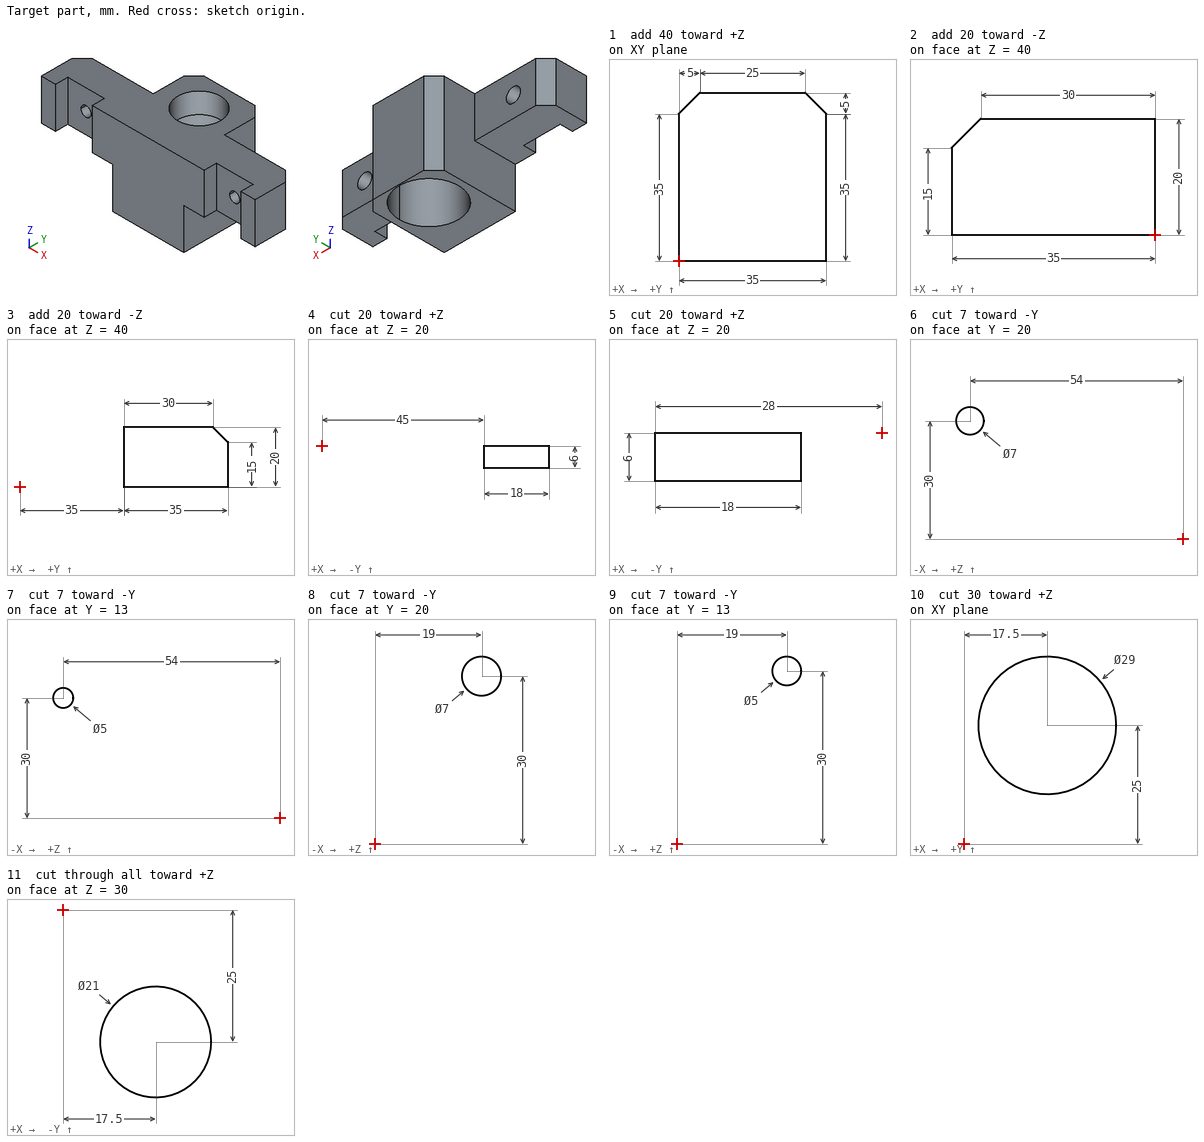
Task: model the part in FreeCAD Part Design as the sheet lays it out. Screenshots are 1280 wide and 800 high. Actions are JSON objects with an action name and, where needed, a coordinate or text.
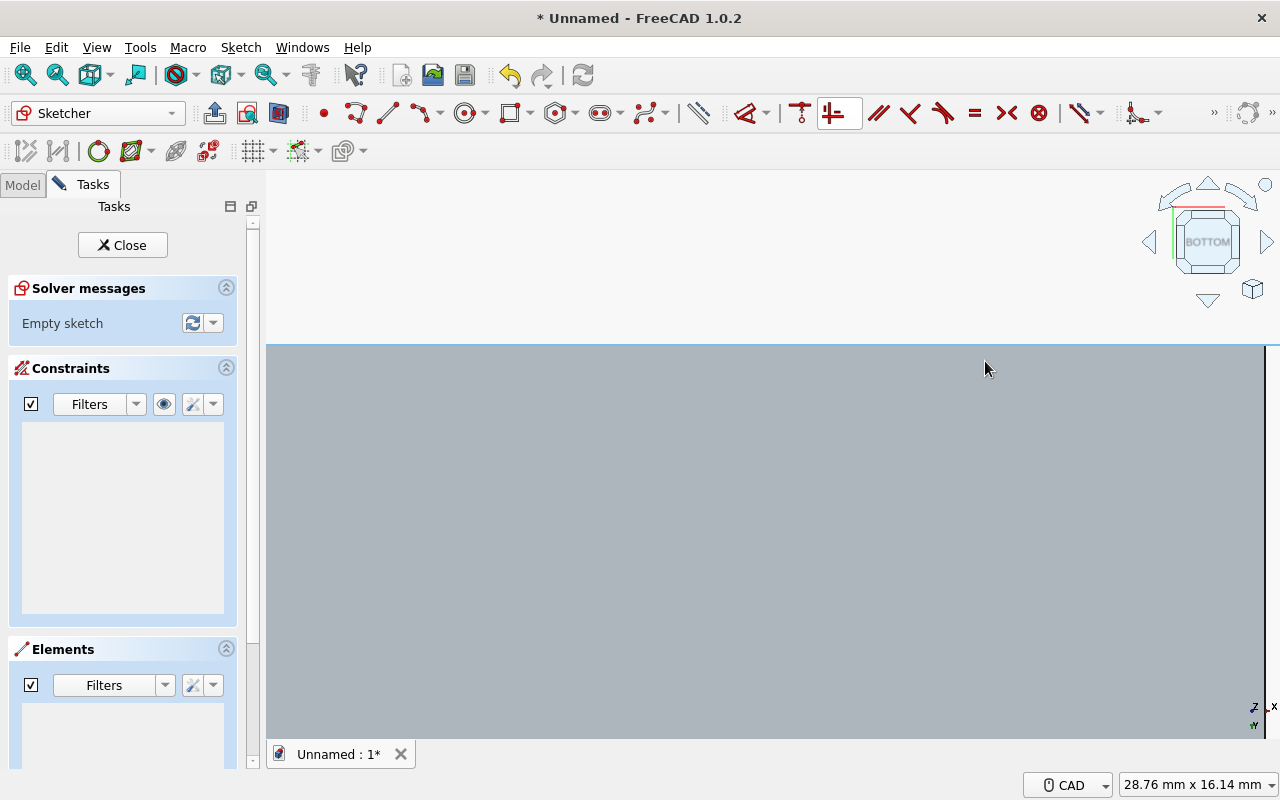
{"action": "left_click", "coordinate": [510, 114]}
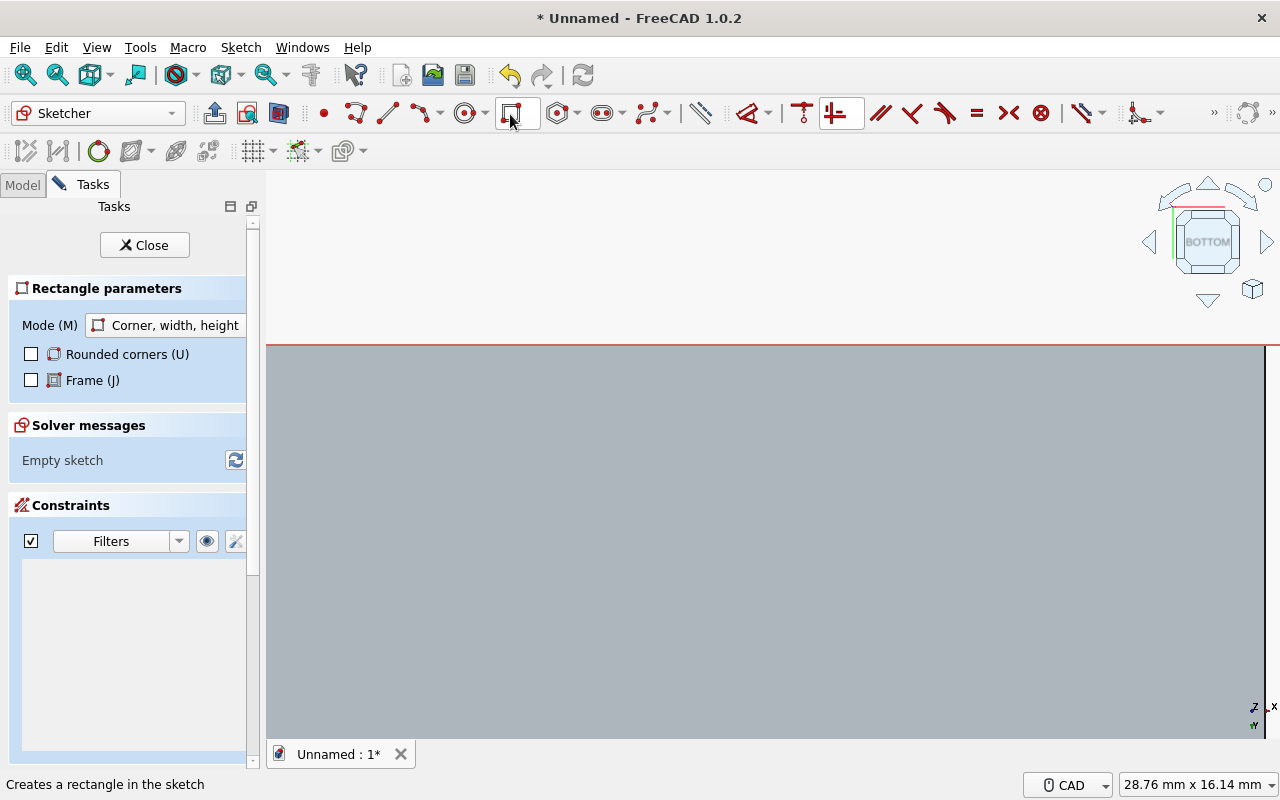
{"action": "left_click", "coordinate": [383, 345]}
{"action": "left_click", "coordinate": [1018, 556]}
{"action": "key", "text": "Escape"}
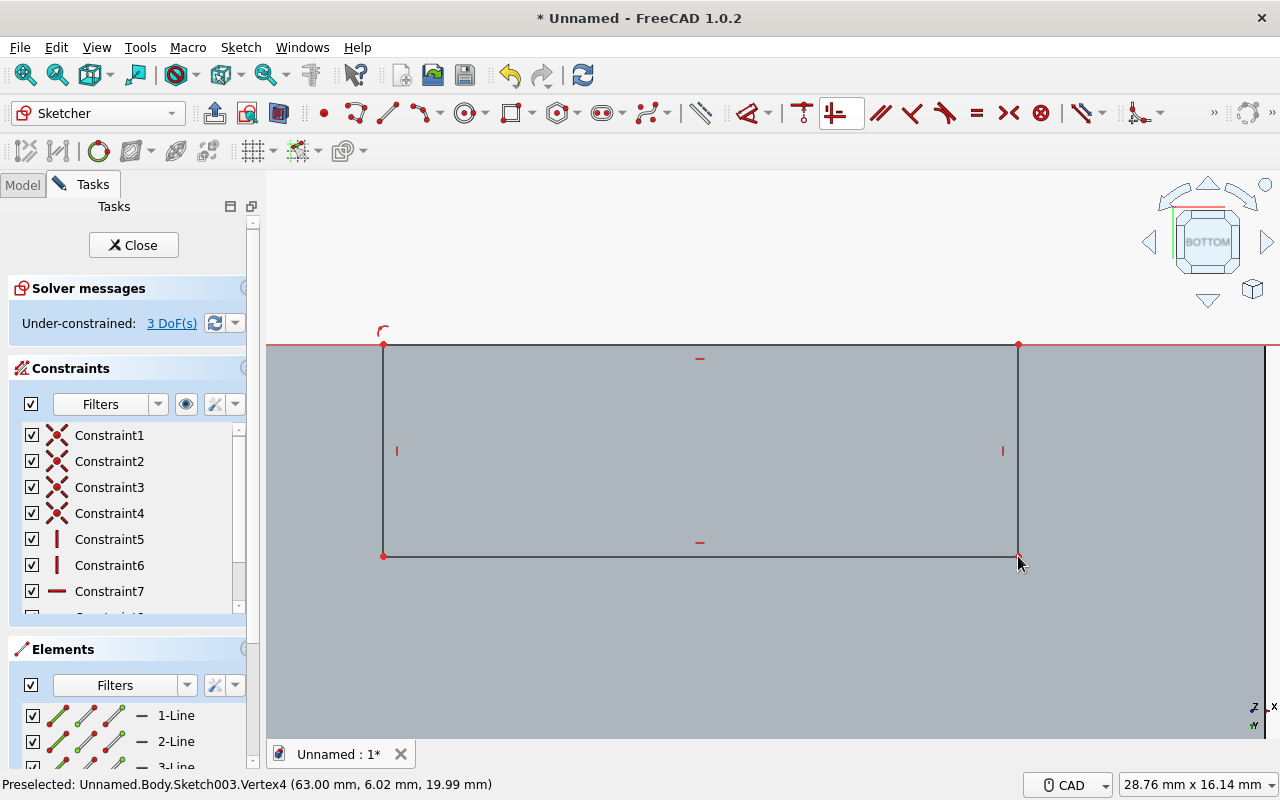
{"action": "left_click", "coordinate": [748, 114]}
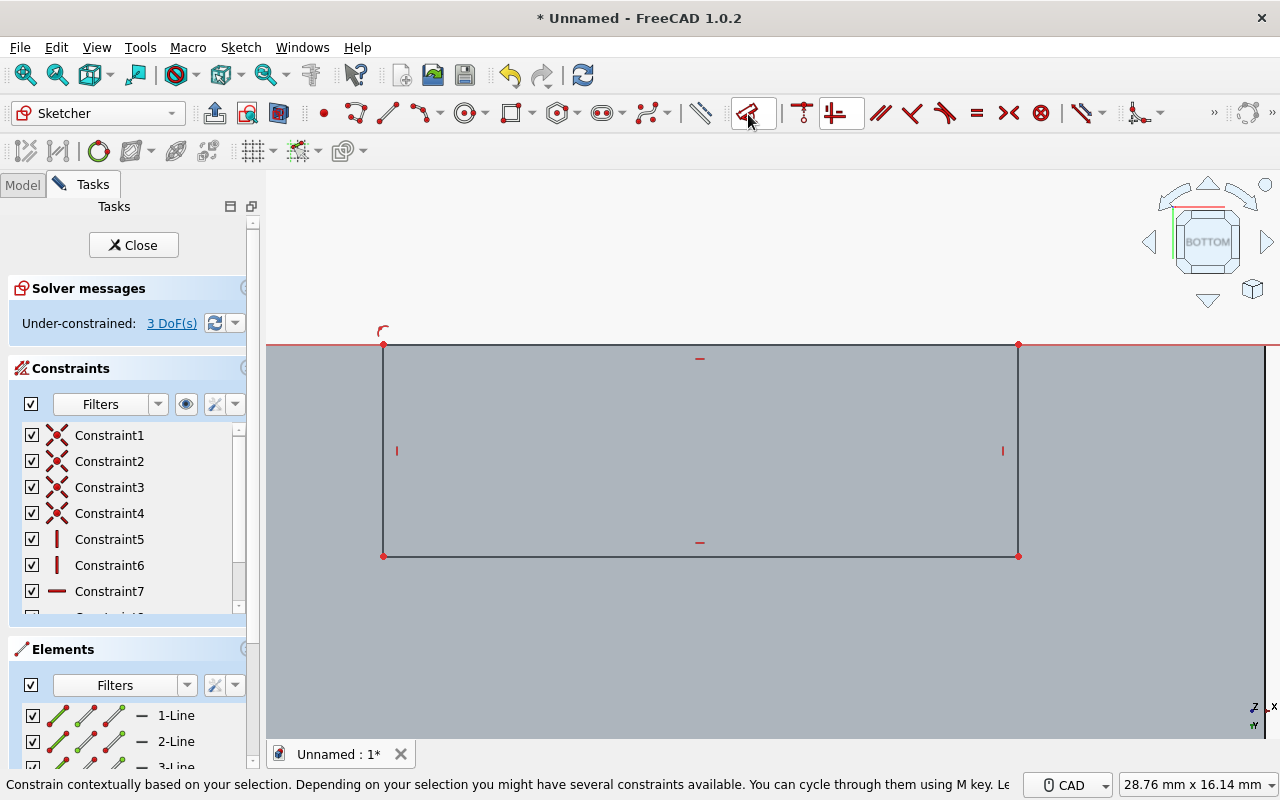
{"action": "left_click", "coordinate": [383, 408]}
{"action": "left_click", "coordinate": [349, 451]}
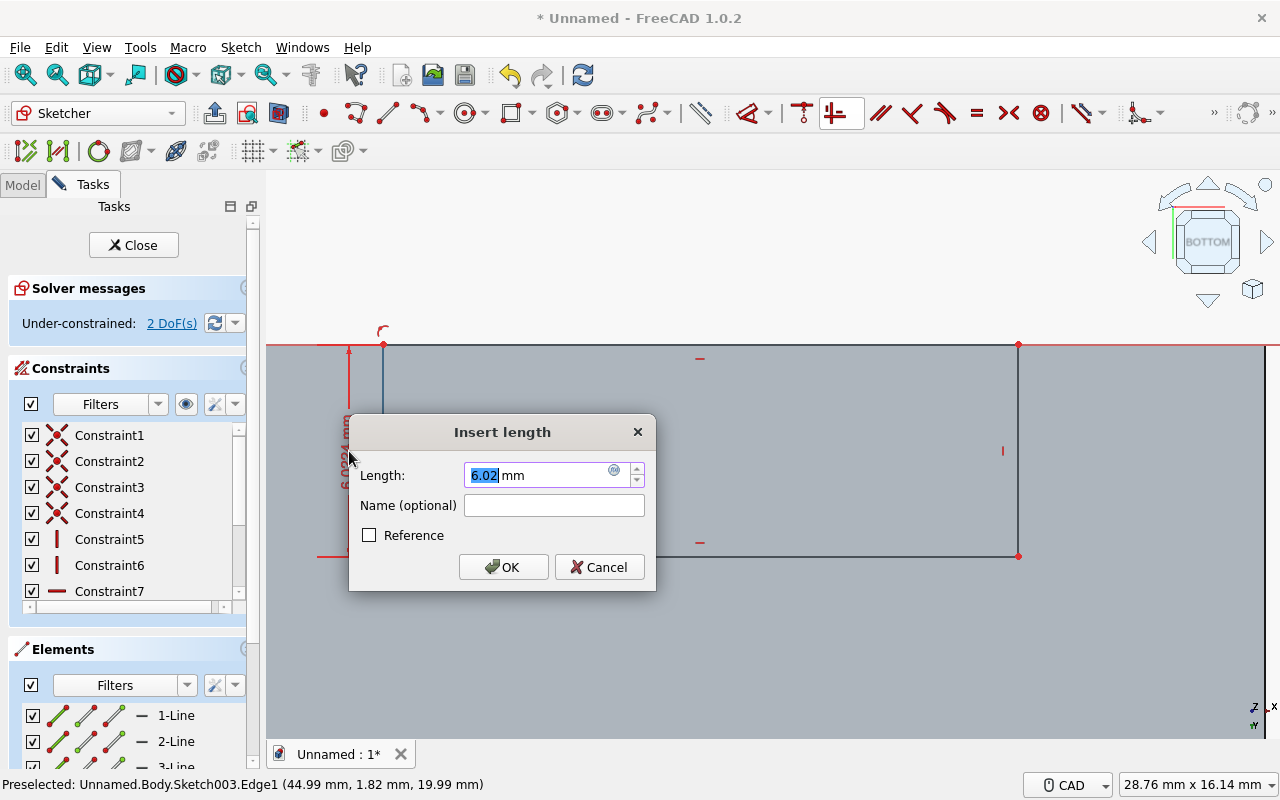
{"action": "type", "text": "6"}
{"action": "key", "text": "Return"}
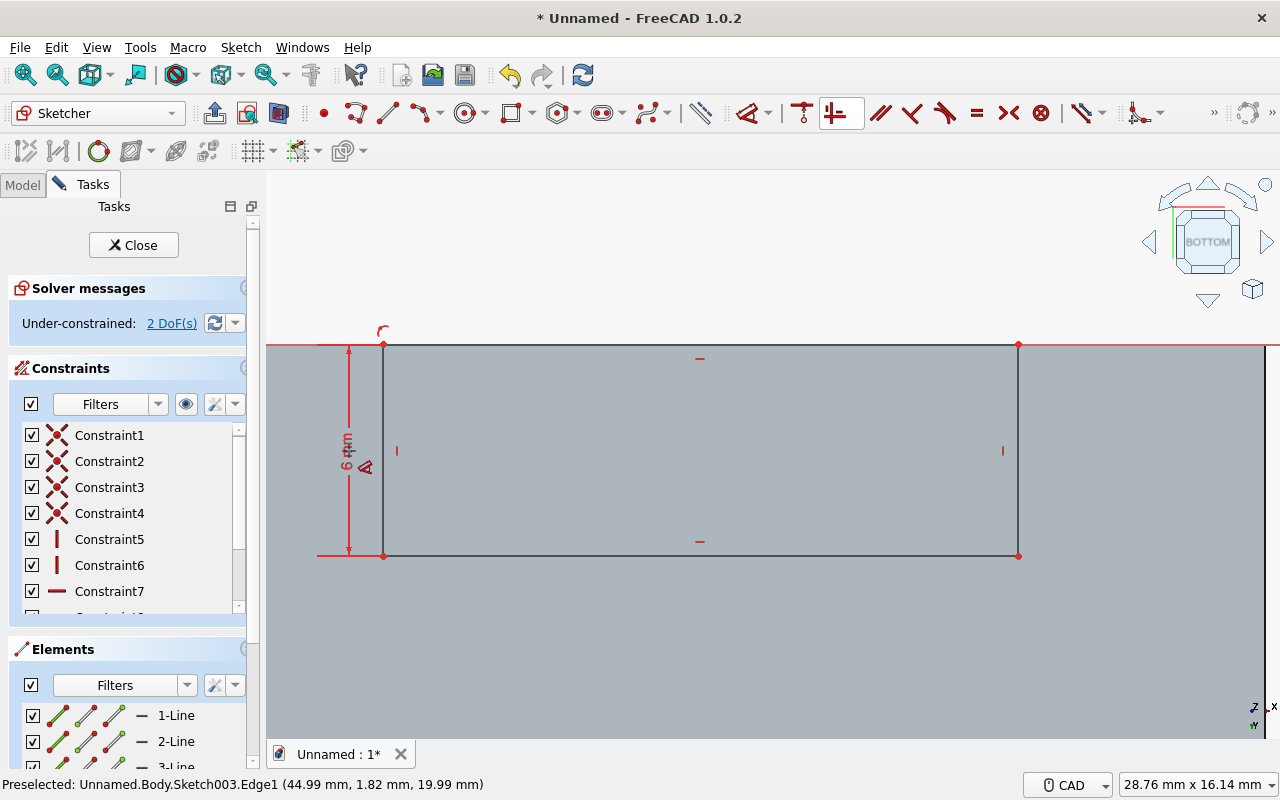
{"action": "left_click", "coordinate": [574, 556]}
{"action": "left_click", "coordinate": [701, 590]}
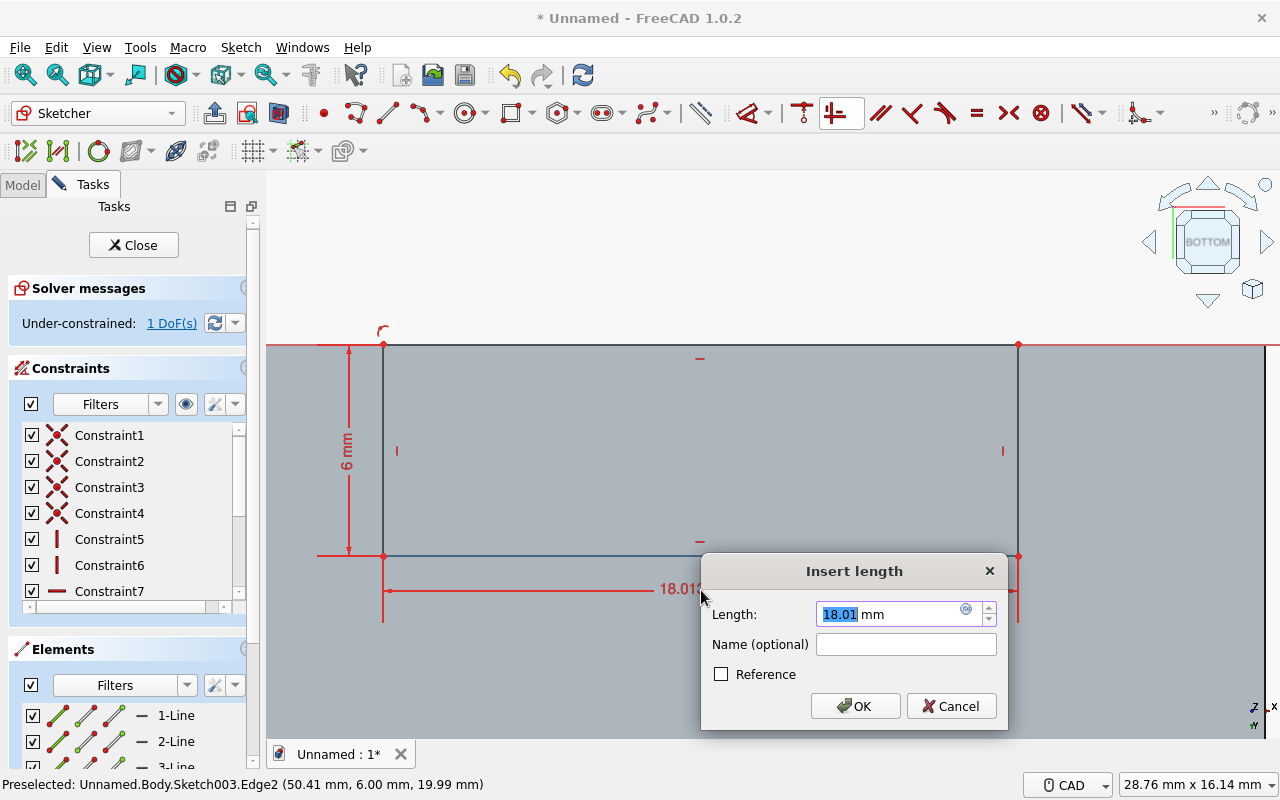
{"action": "type", "text": "18"}
{"action": "key", "text": "Return"}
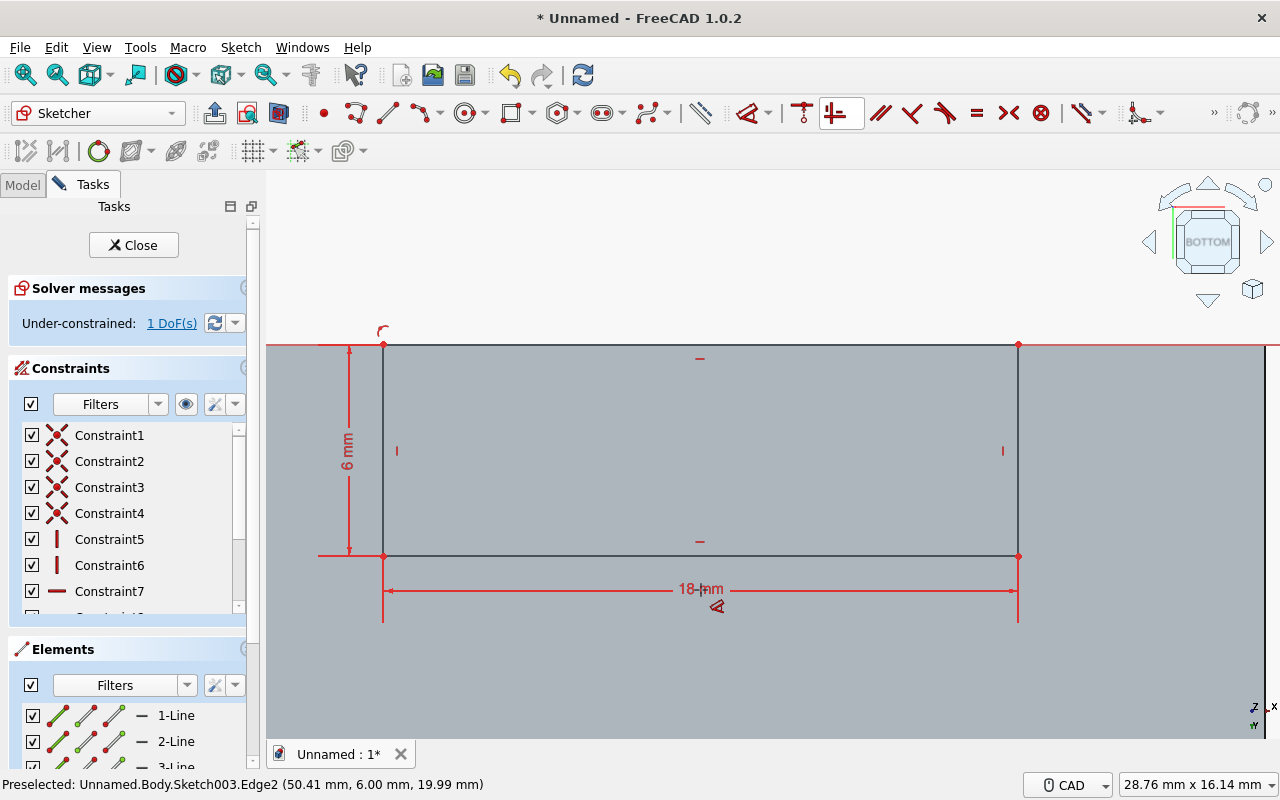
{"action": "left_click", "coordinate": [383, 345]}
{"action": "left_click", "coordinate": [339, 311]}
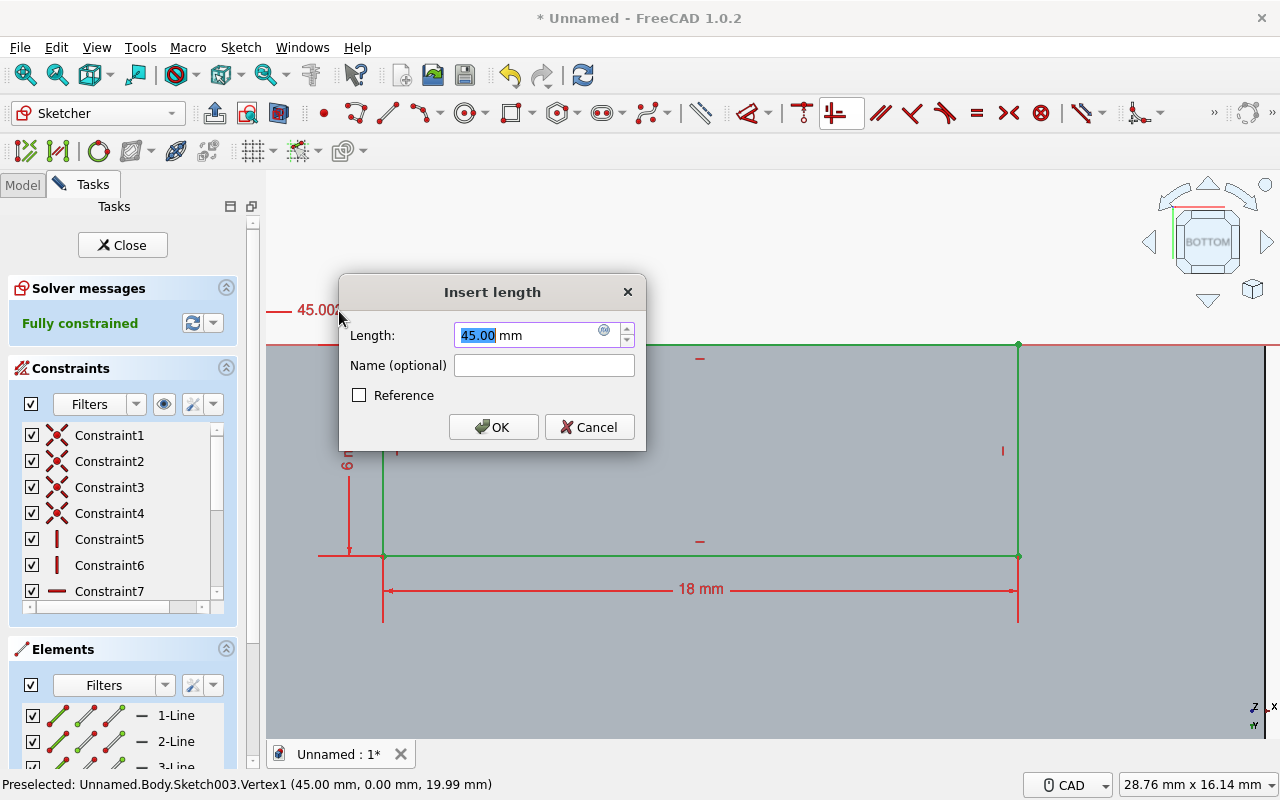
{"action": "type", "text": "45"}
{"action": "key", "text": "Return"}
{"action": "key", "text": "Escape"}